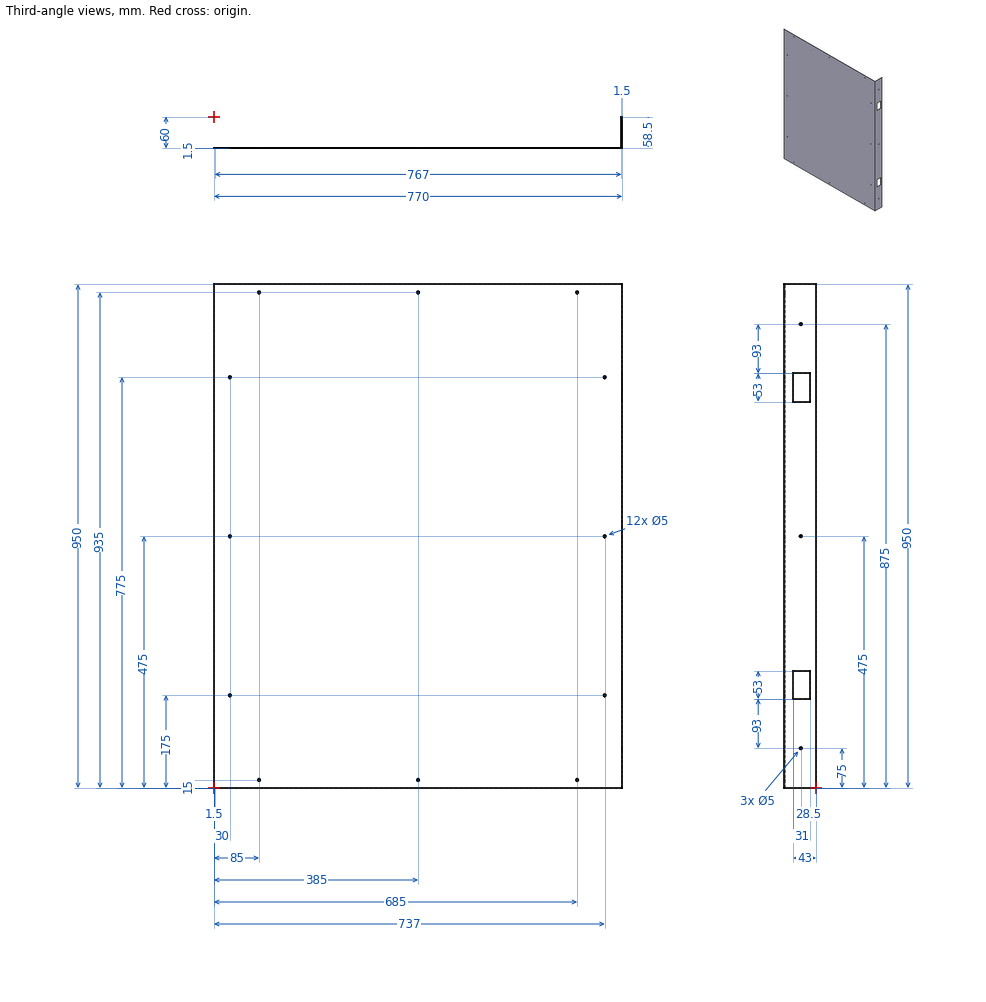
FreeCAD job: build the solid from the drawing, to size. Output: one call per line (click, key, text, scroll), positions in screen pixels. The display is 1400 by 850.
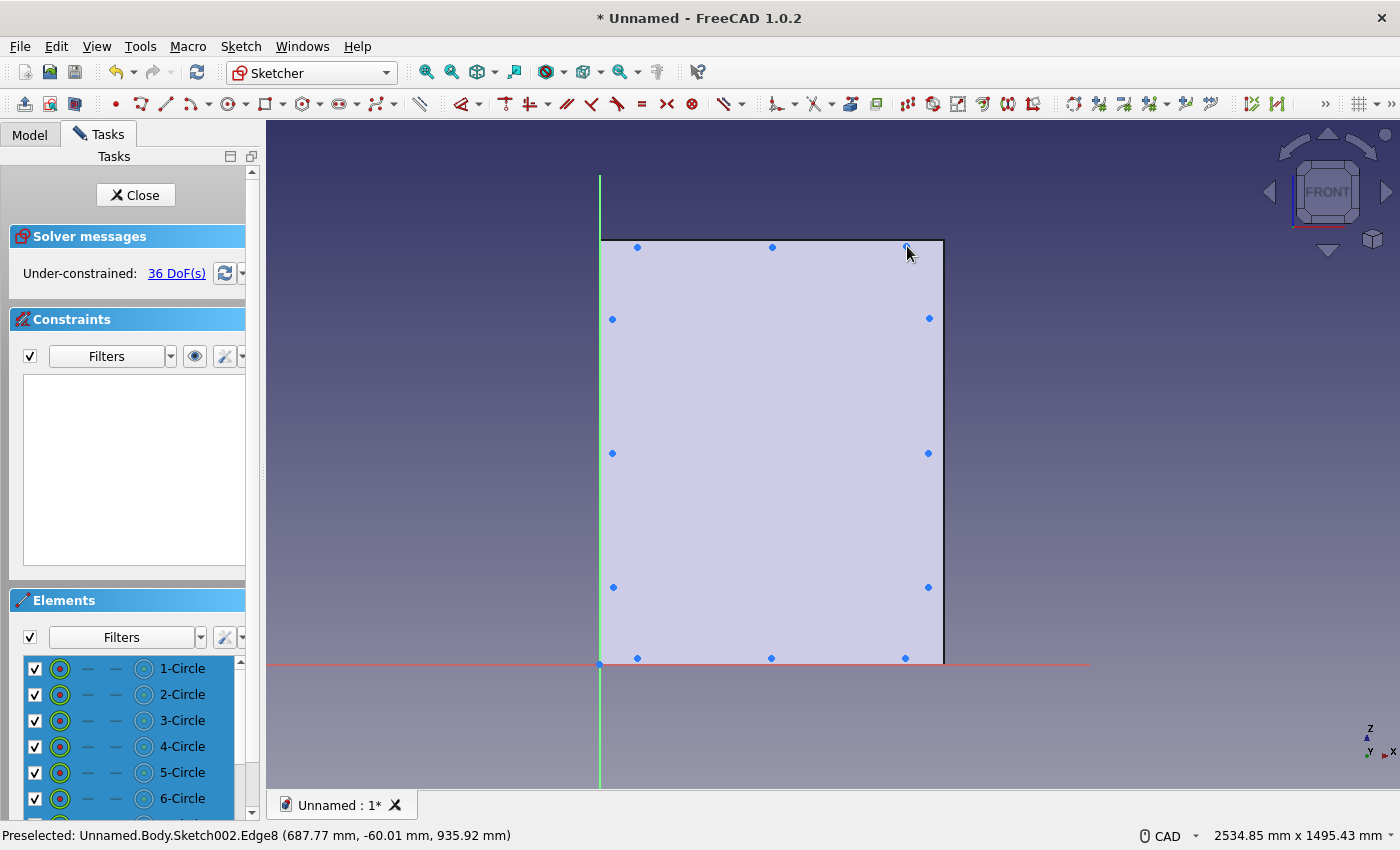
scroll(639, 246, up, 11)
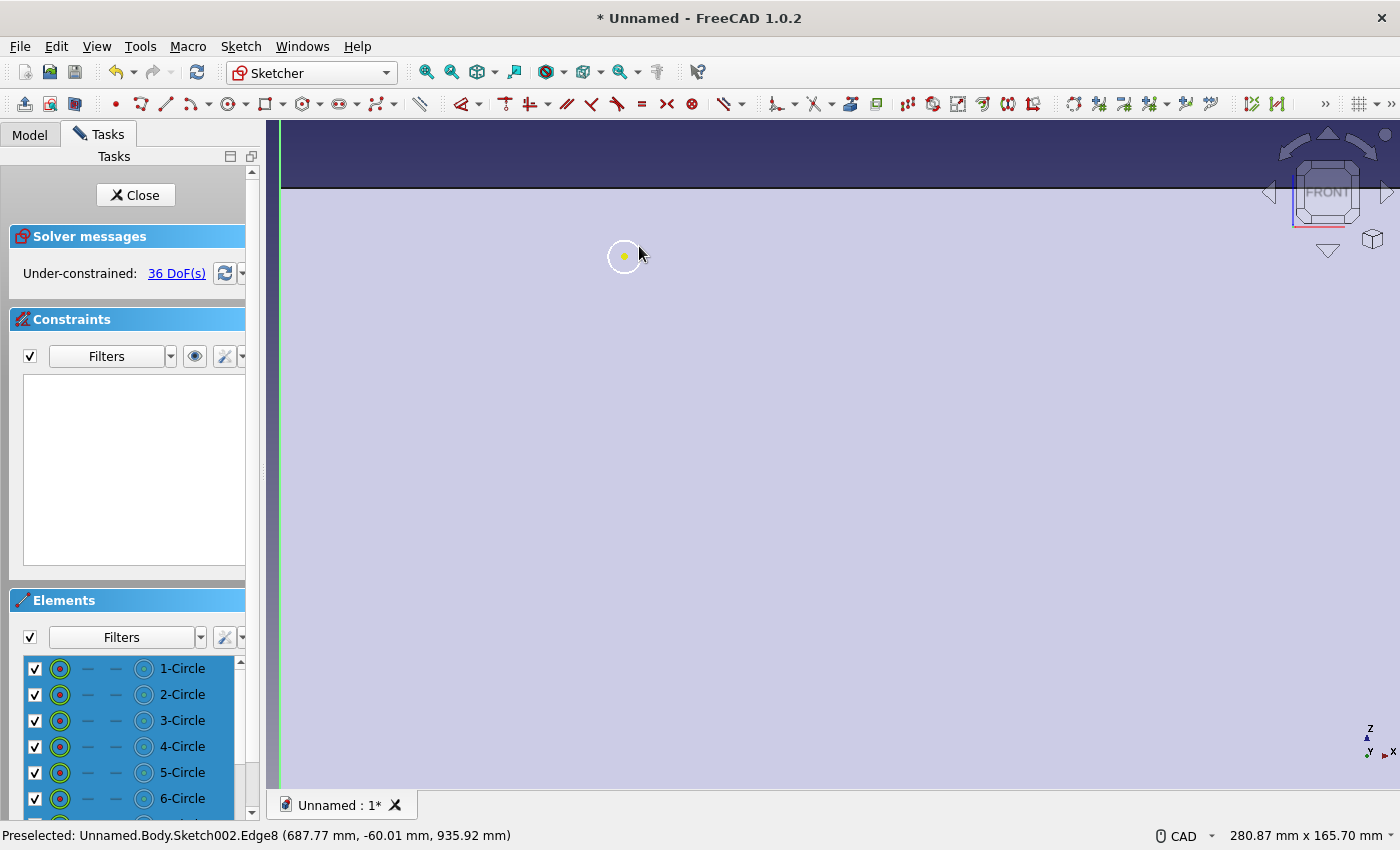
click(636, 245)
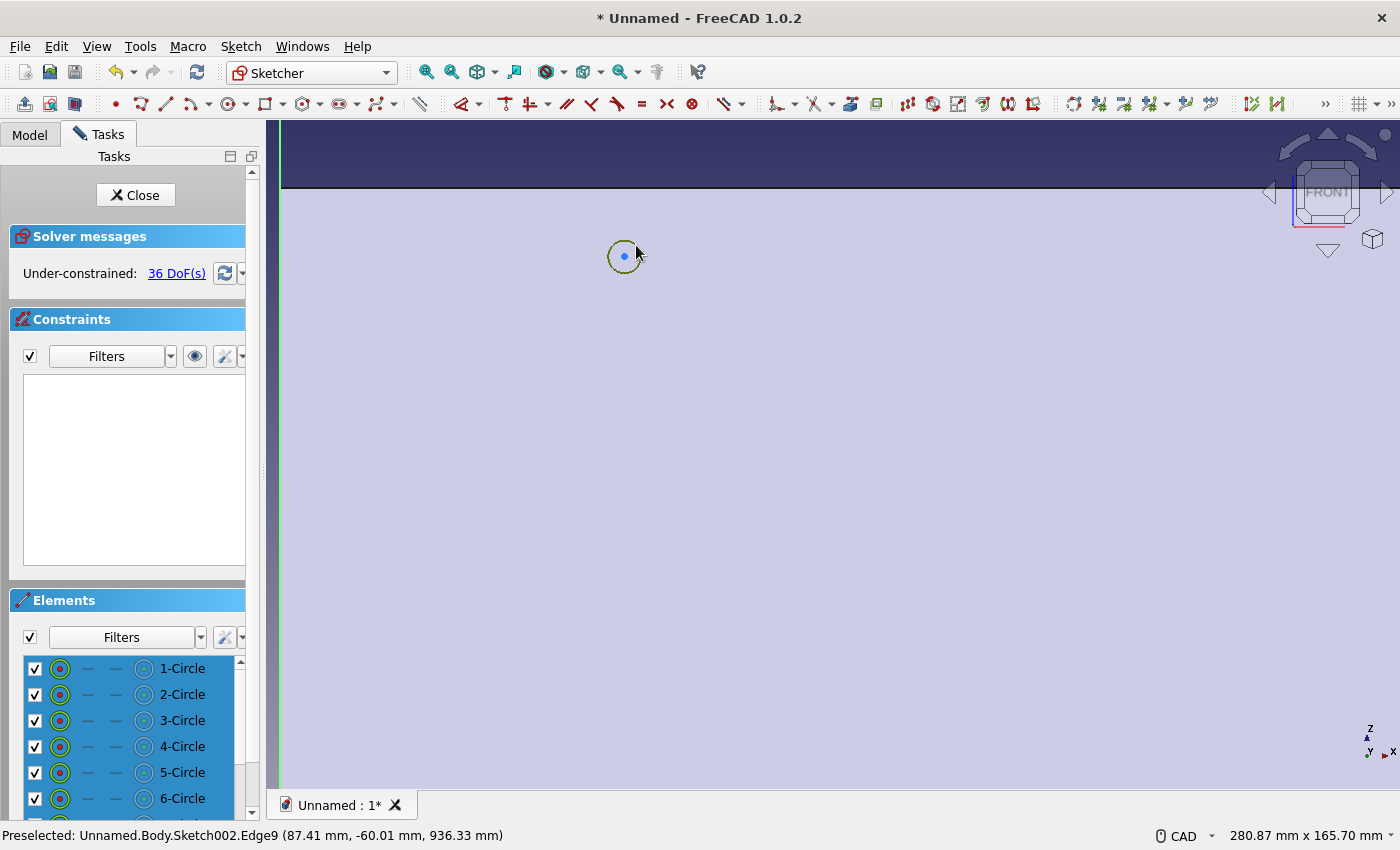
scroll(639, 246, down, 11)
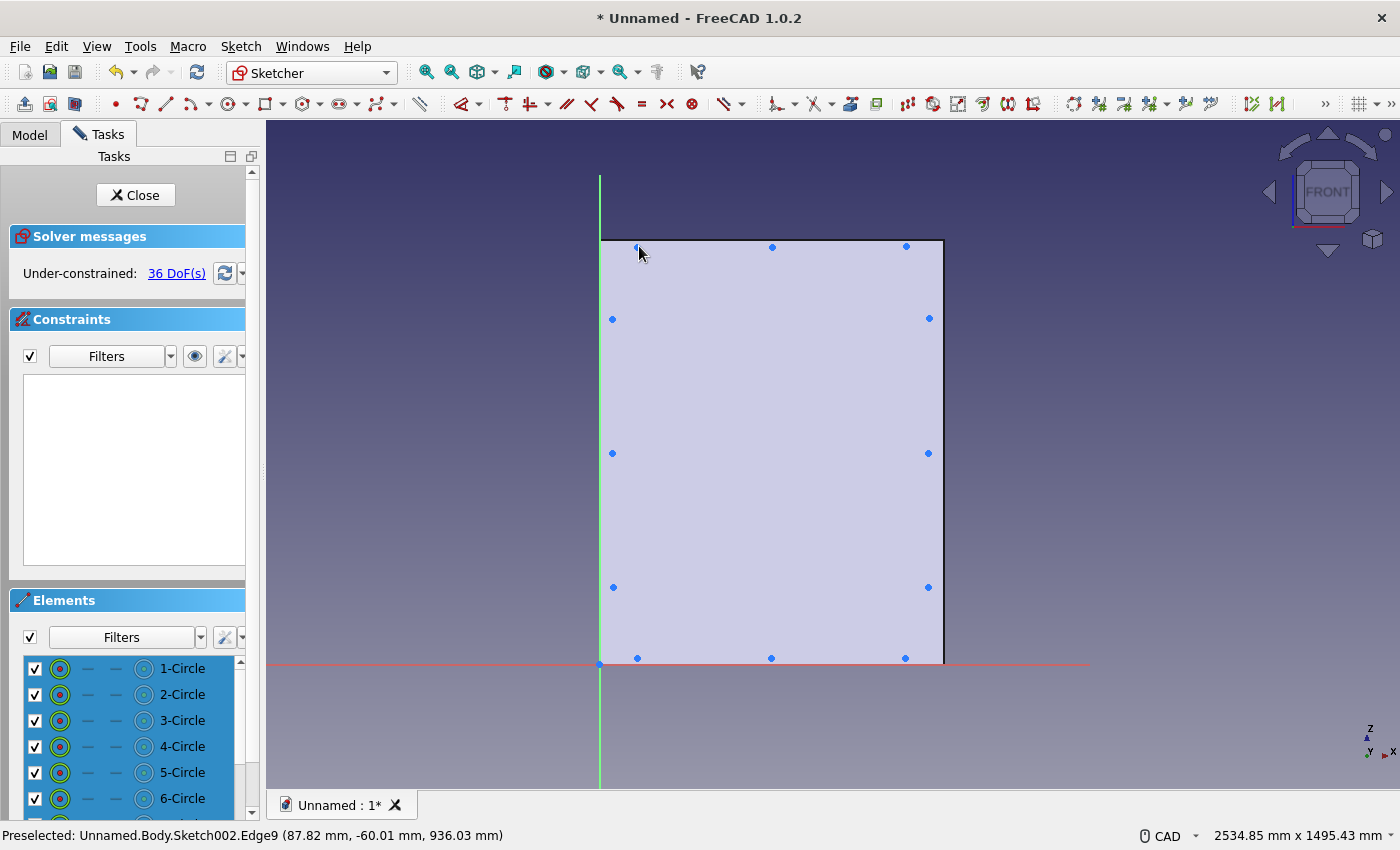
scroll(639, 657, up, 12)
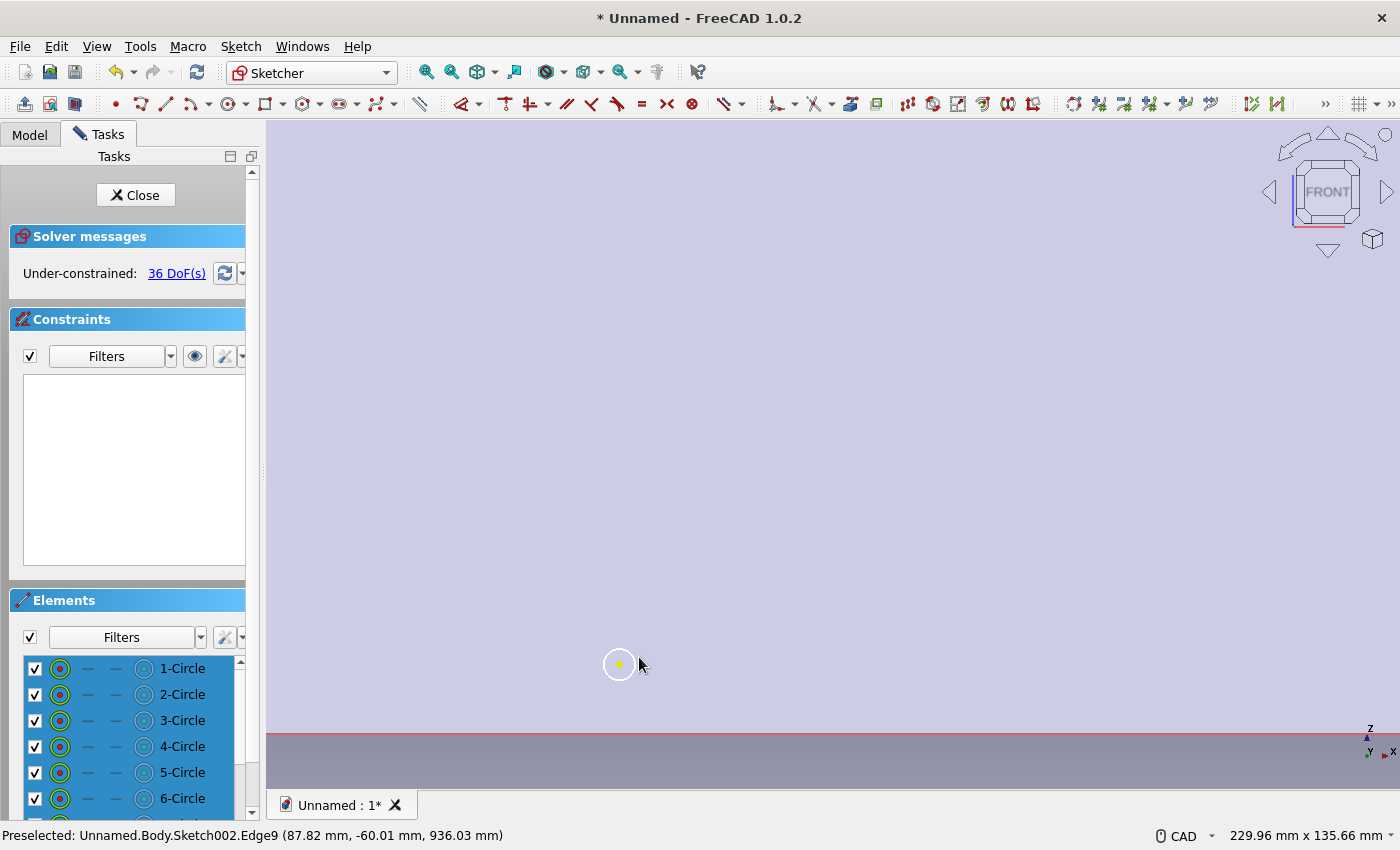
click(630, 654)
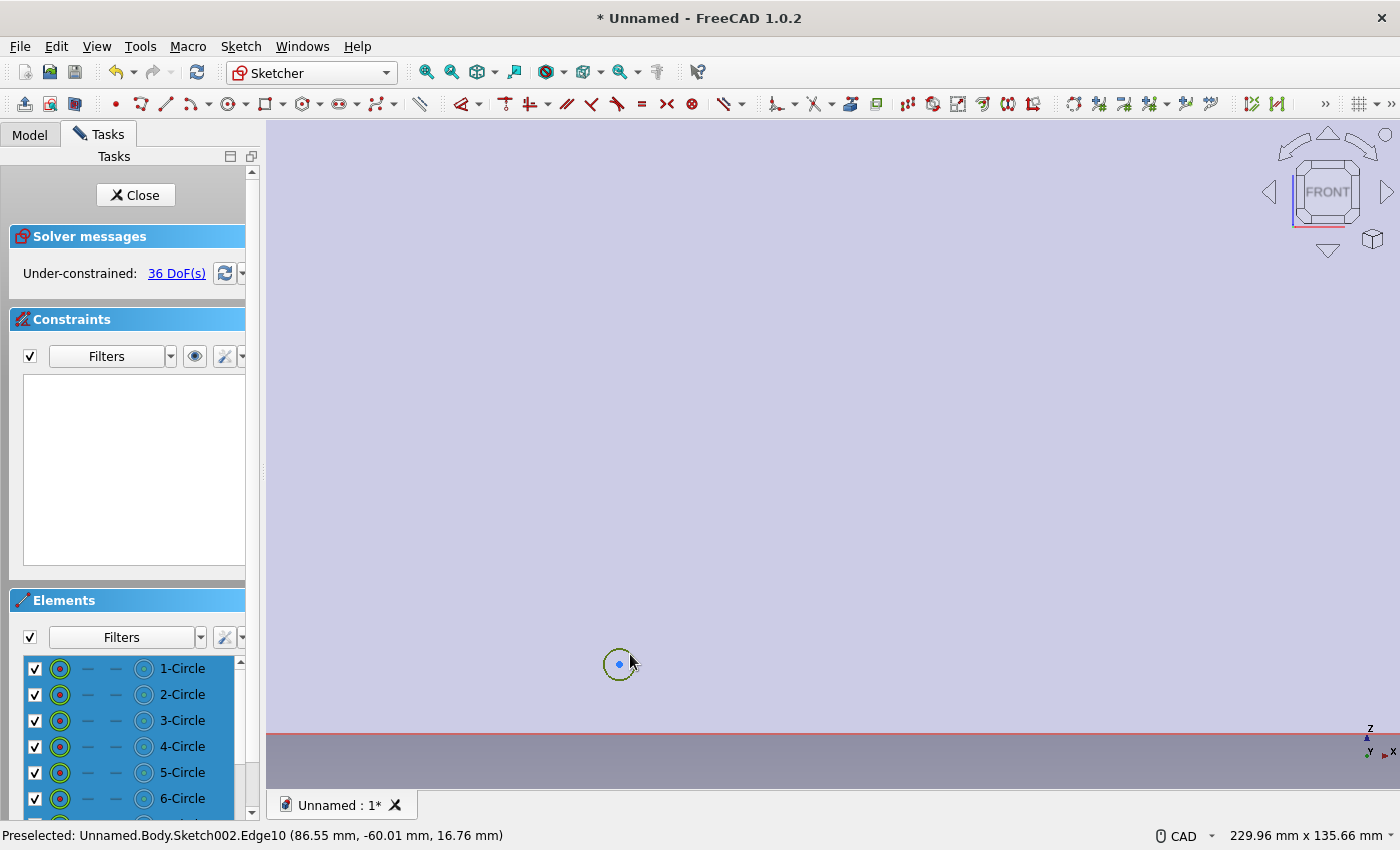
scroll(639, 657, down, 12)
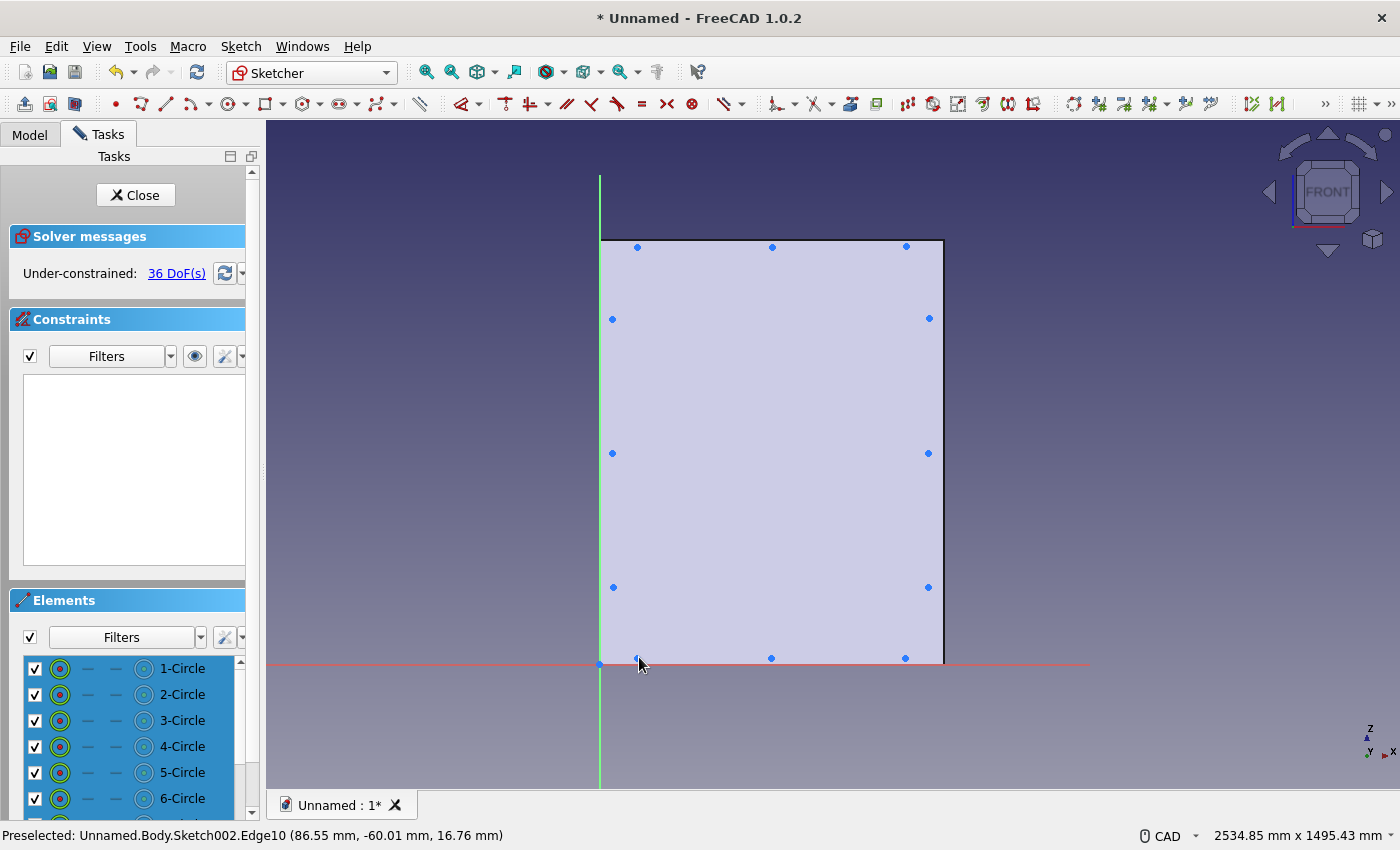
scroll(907, 657, up, 12)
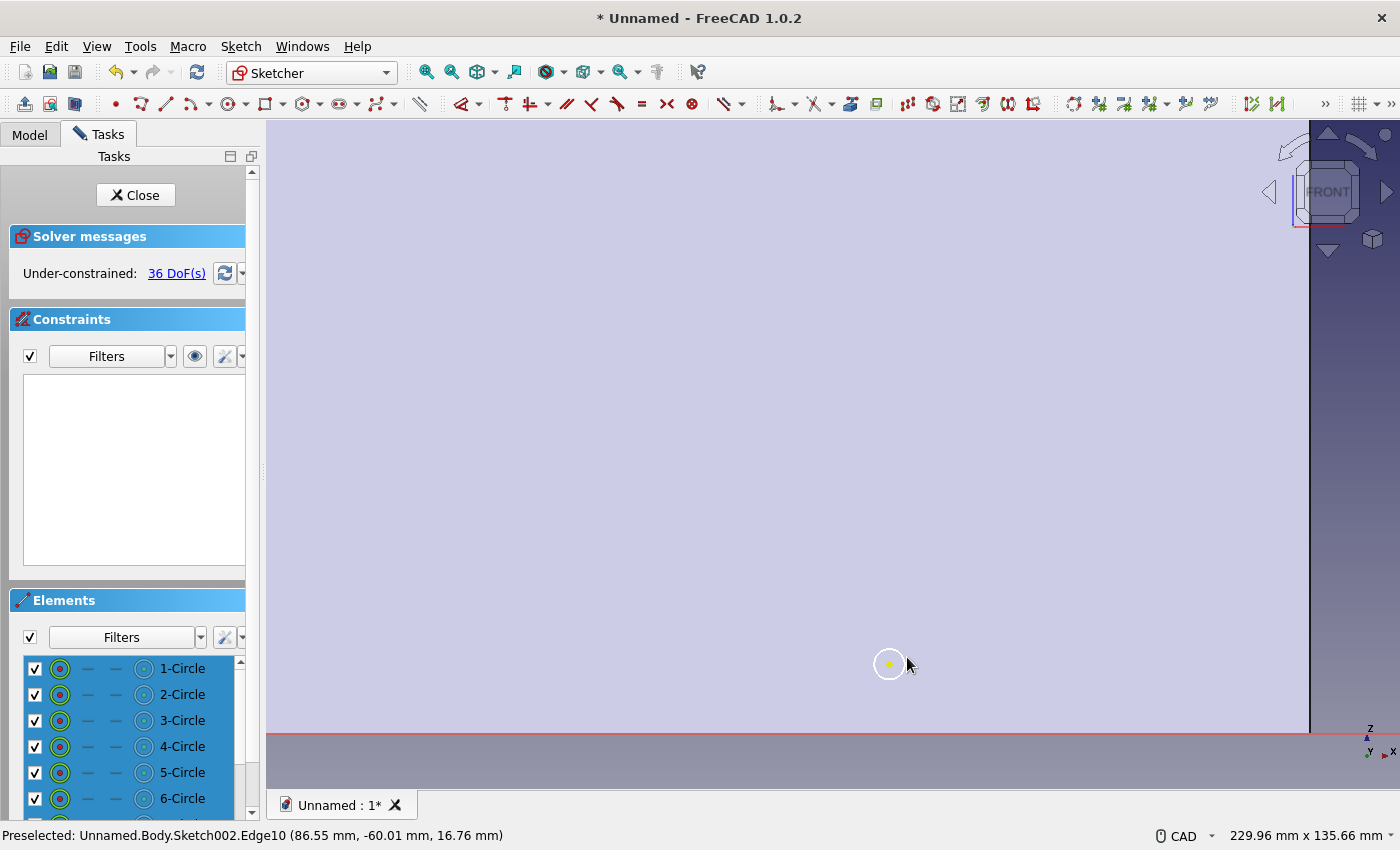
click(900, 654)